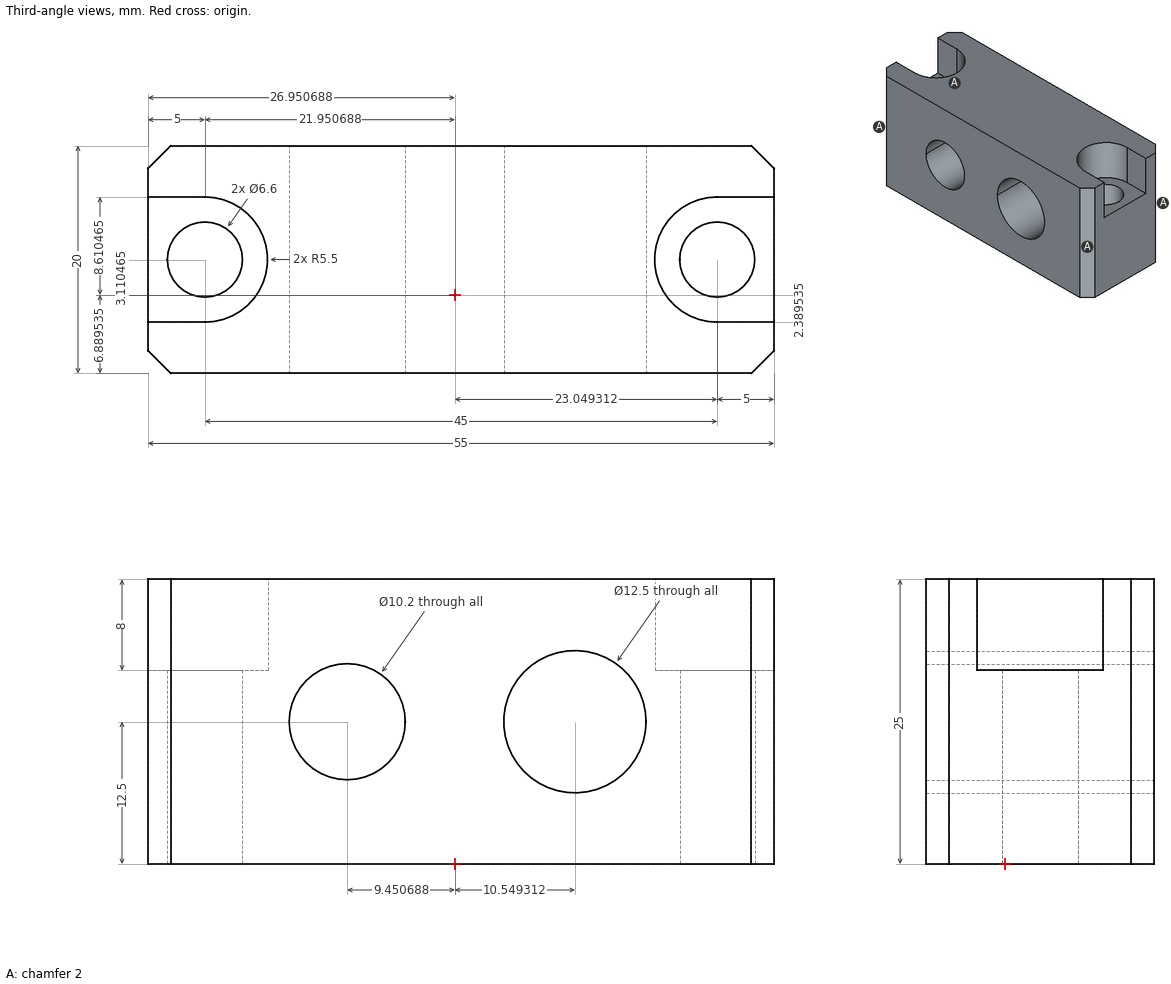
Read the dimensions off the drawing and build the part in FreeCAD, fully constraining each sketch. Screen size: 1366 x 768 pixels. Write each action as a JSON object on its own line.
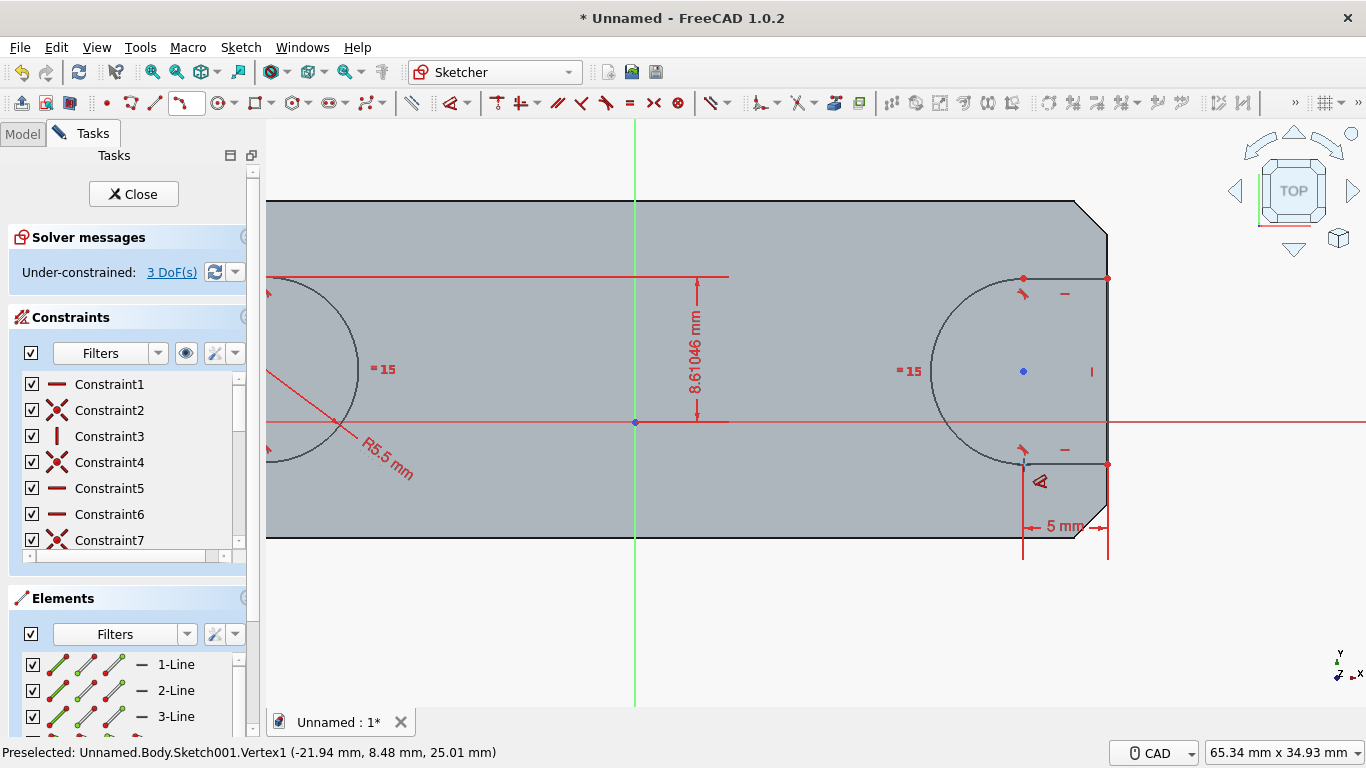
{"action": "left_click", "coordinate": [1023, 464]}
{"action": "left_click", "coordinate": [1057, 443]}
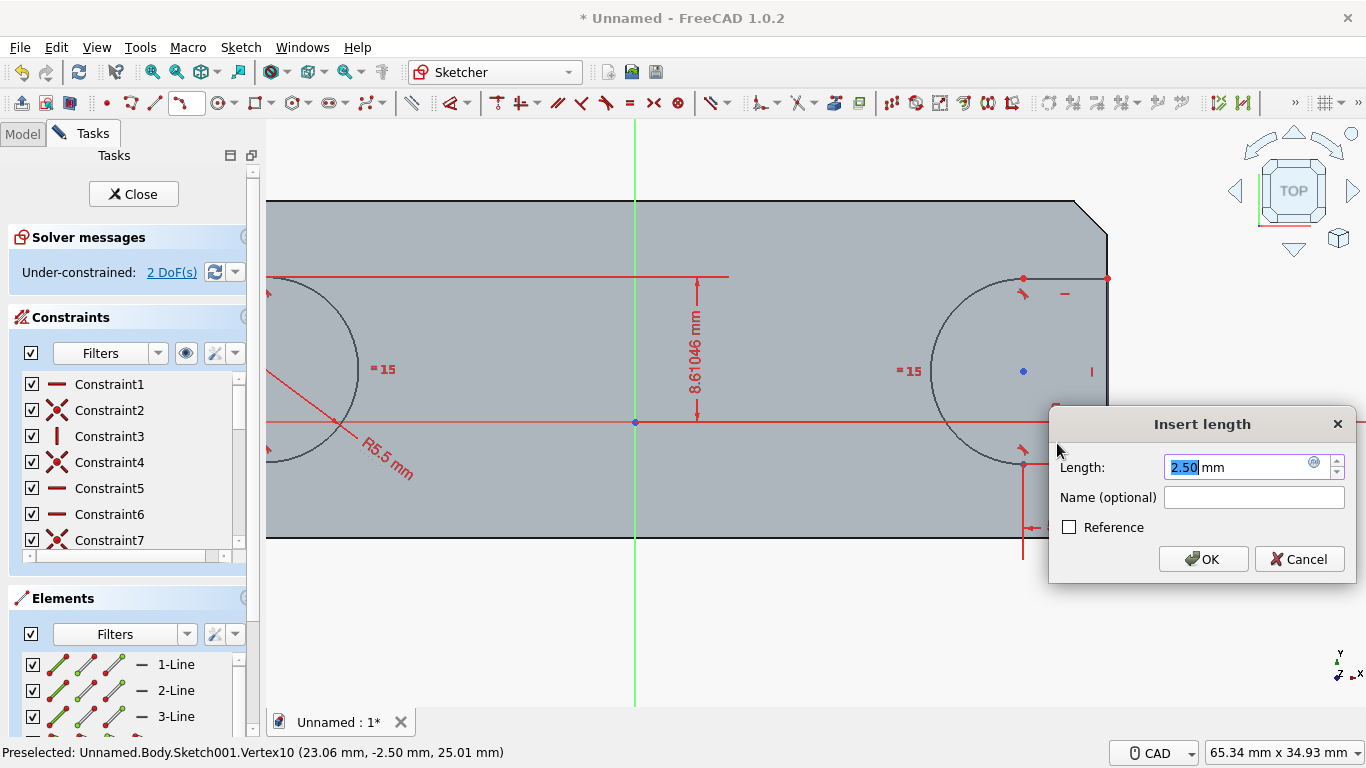
{"action": "type", "text": "2.389535"}
{"action": "key", "text": "Return"}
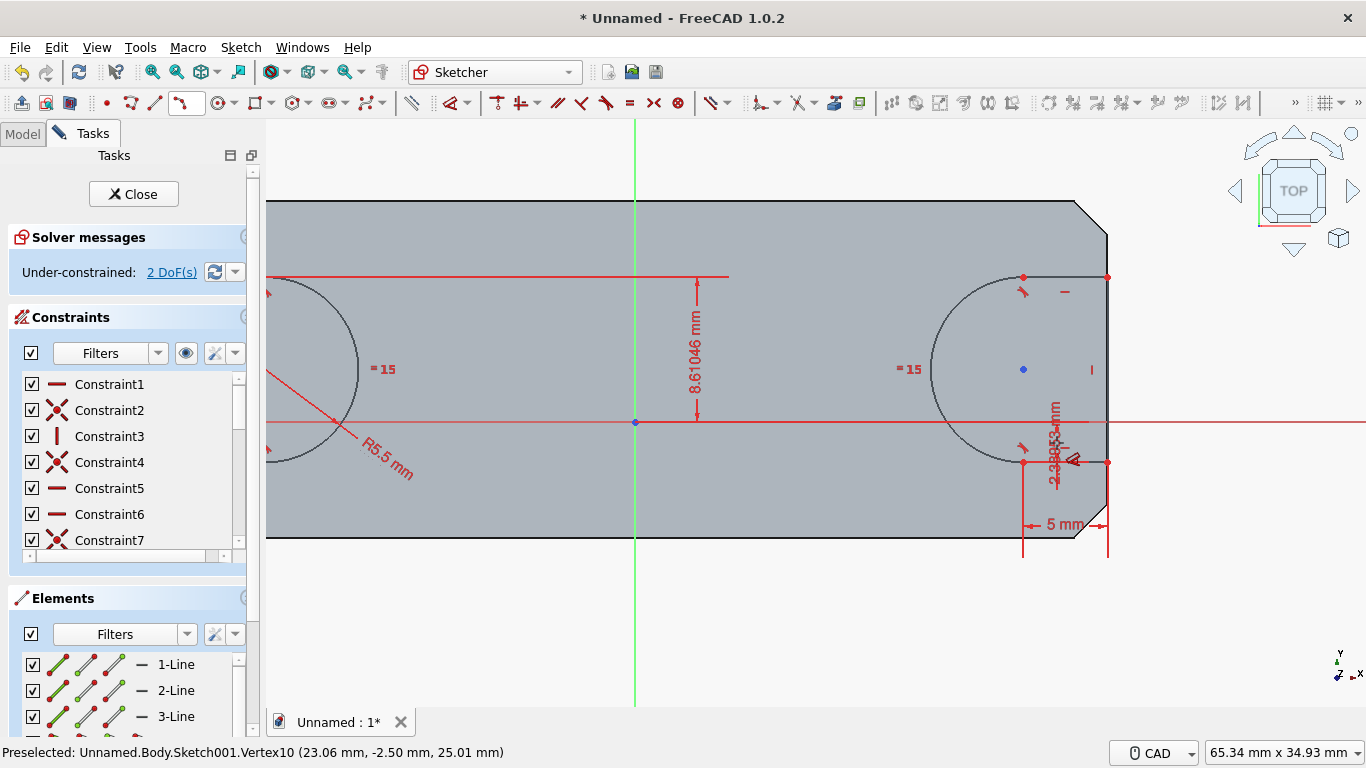
{"action": "scroll", "coordinate": [957, 501], "scroll_direction": "down", "scroll_amount": 2}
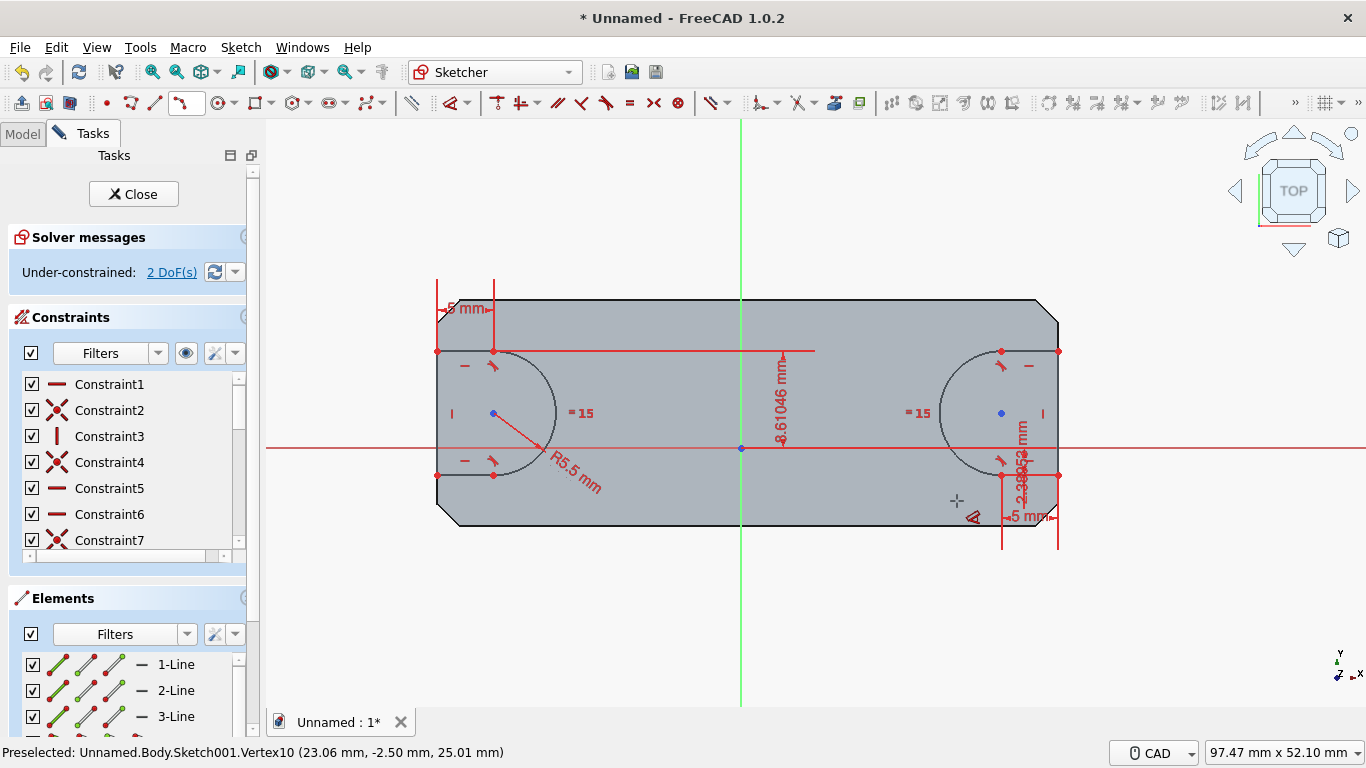
{"action": "left_click", "coordinate": [494, 351]}
{"action": "left_click", "coordinate": [618, 317]}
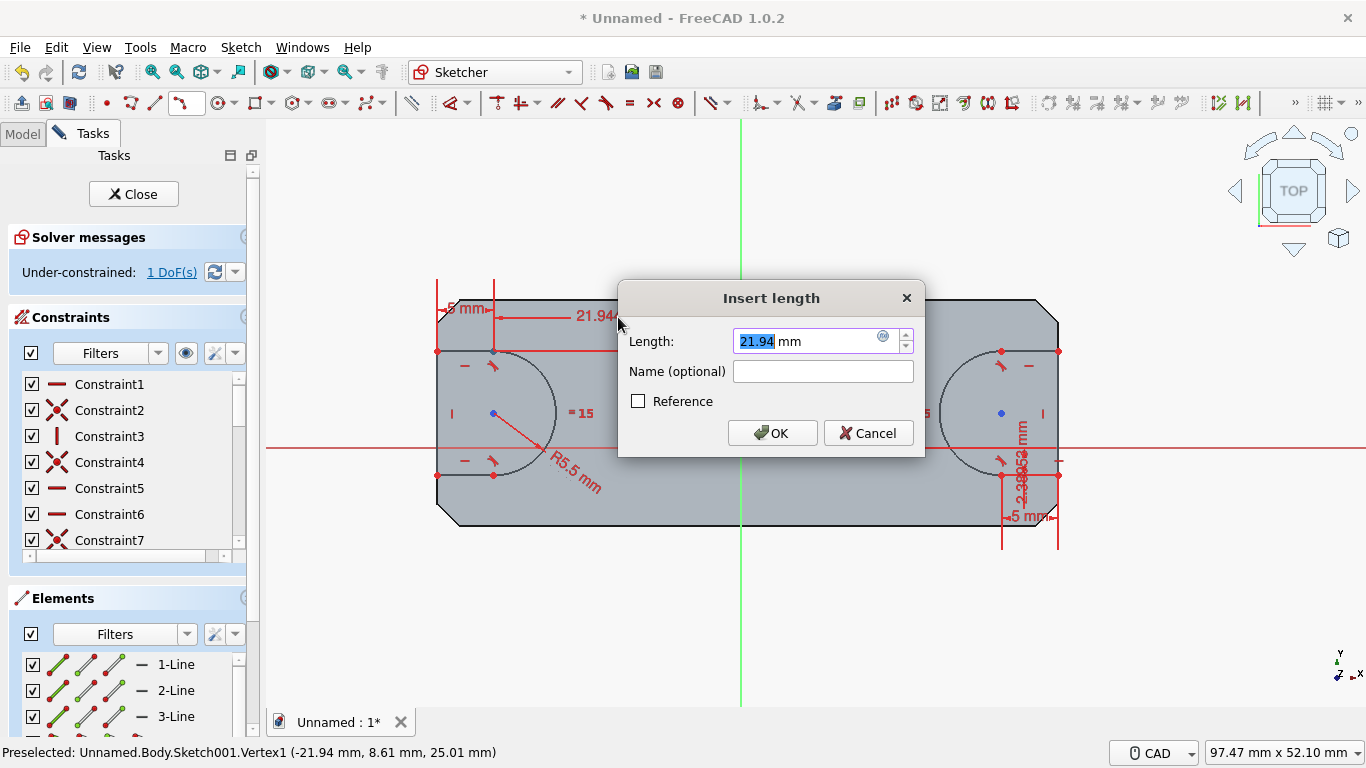
{"action": "type", "text": "21.950688"}
{"action": "key", "text": "Return"}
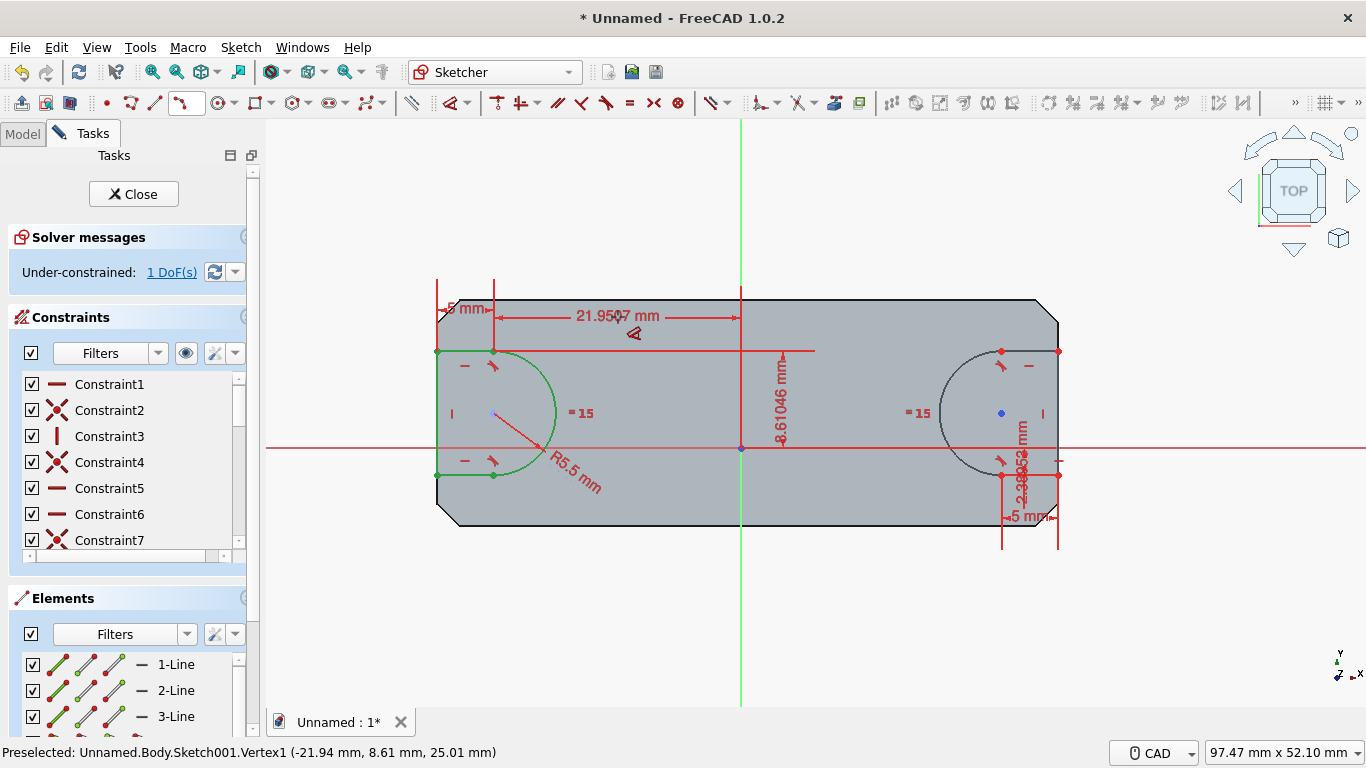
{"action": "left_click", "coordinate": [1002, 475]}
{"action": "left_click", "coordinate": [872, 509]}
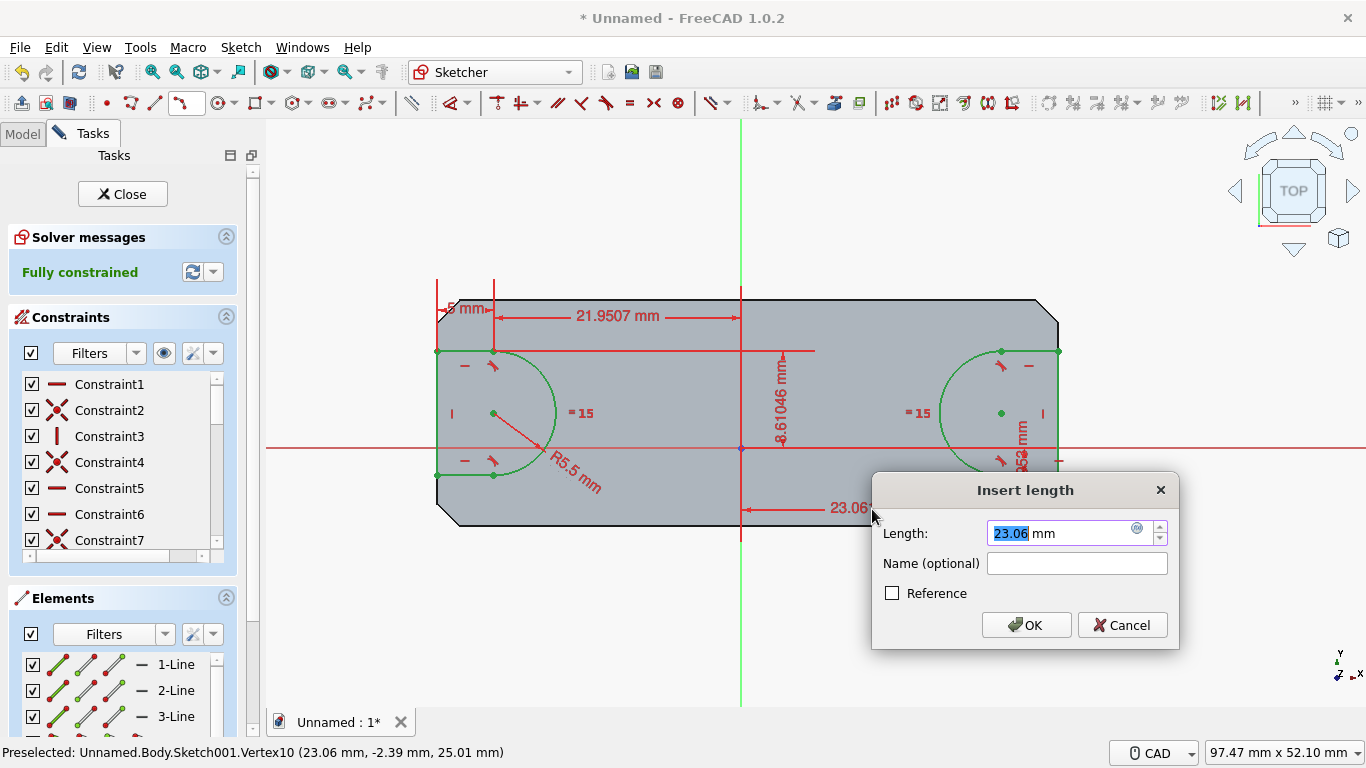
{"action": "type", "text": "23.049312"}
{"action": "key", "text": "Return"}
{"action": "key", "text": "Escape"}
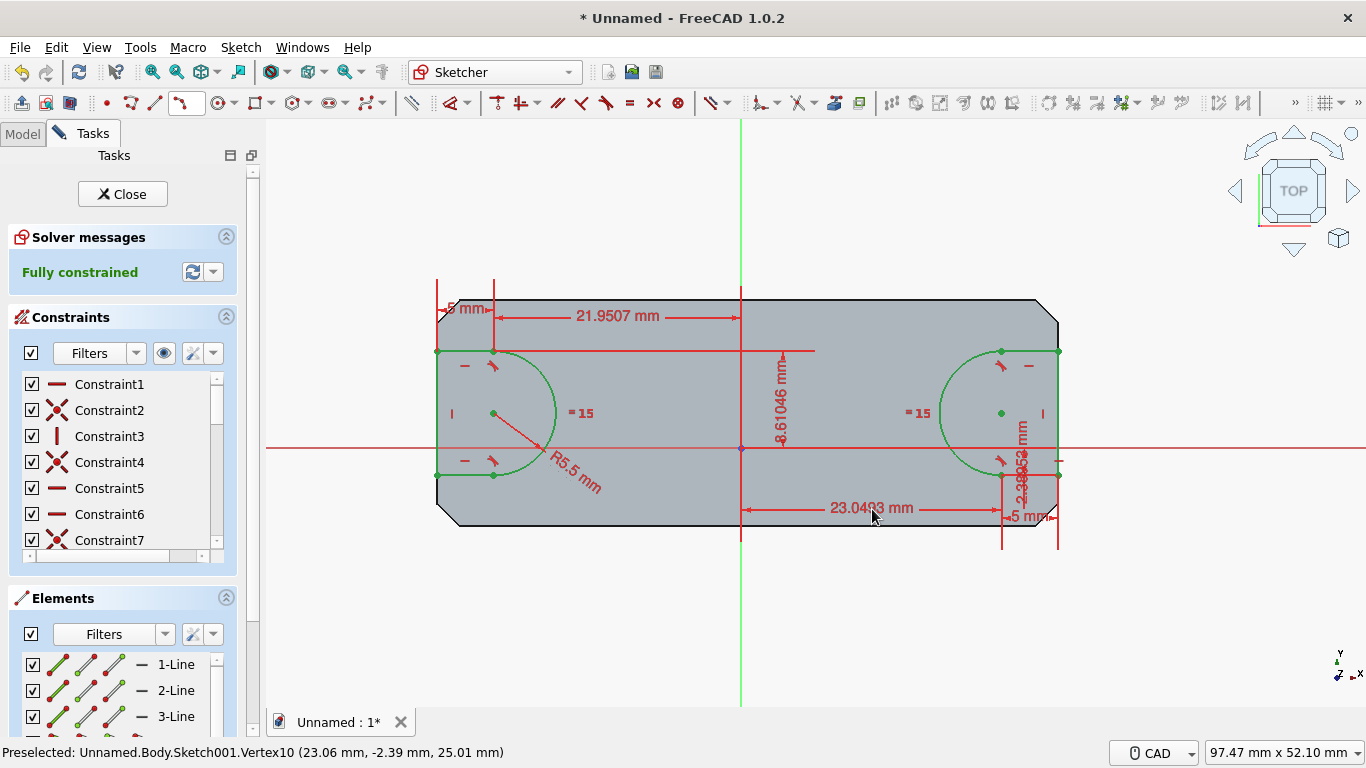
{"action": "left_click", "coordinate": [123, 194]}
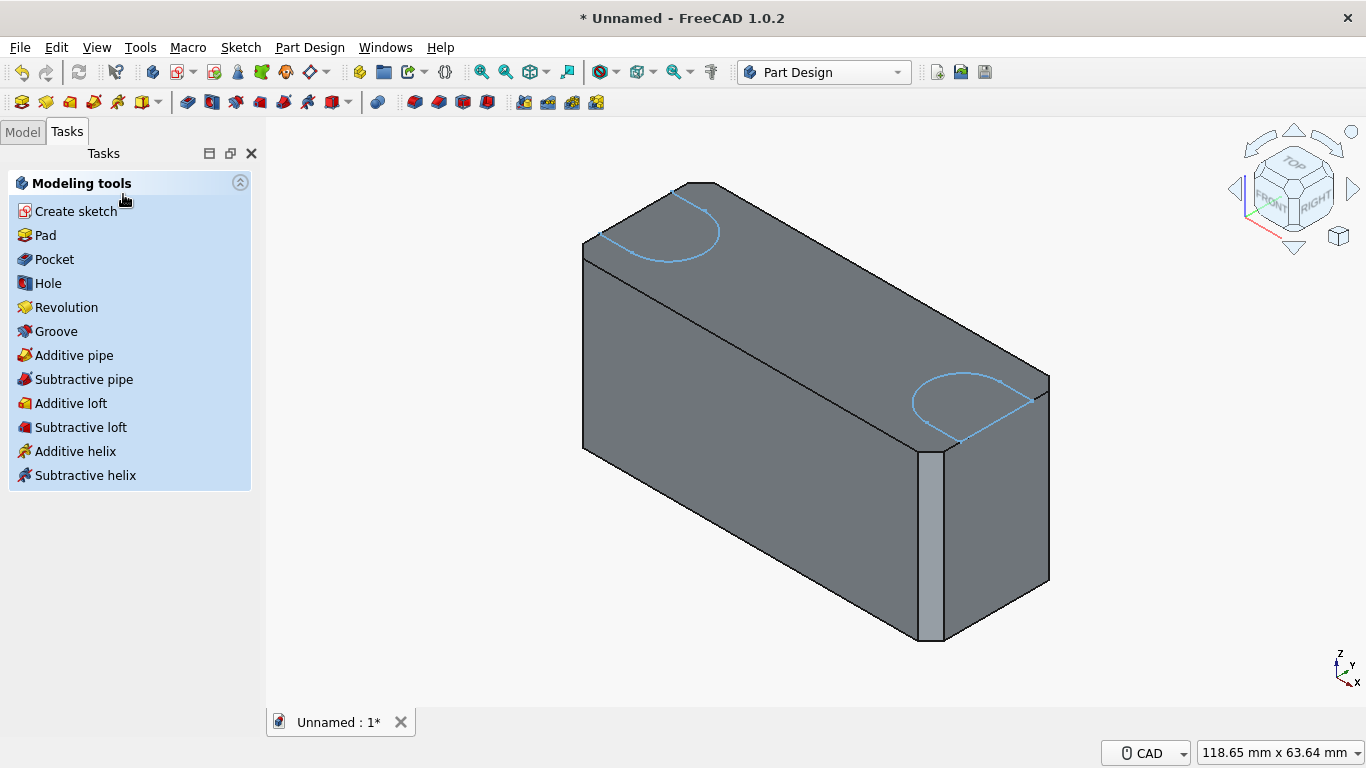
{"action": "left_click", "coordinate": [188, 102]}